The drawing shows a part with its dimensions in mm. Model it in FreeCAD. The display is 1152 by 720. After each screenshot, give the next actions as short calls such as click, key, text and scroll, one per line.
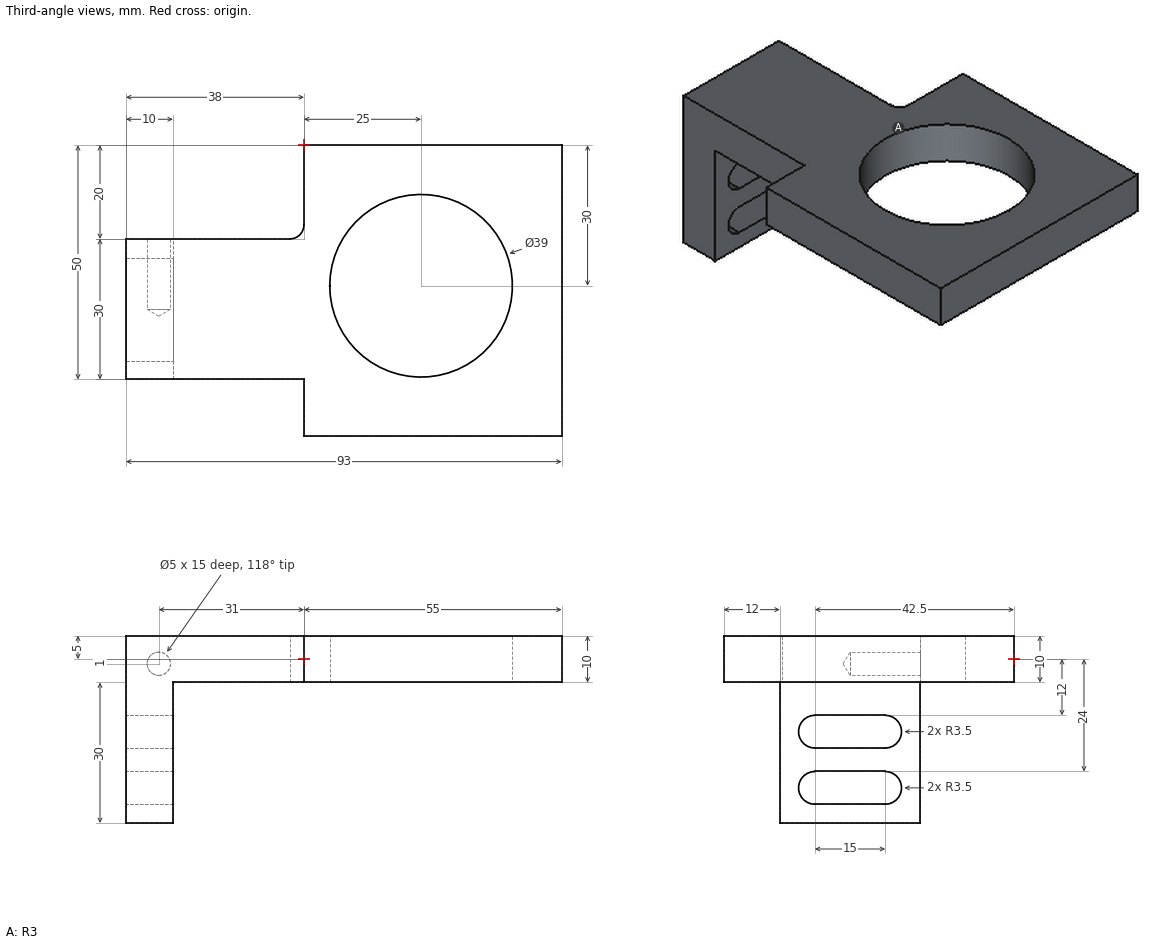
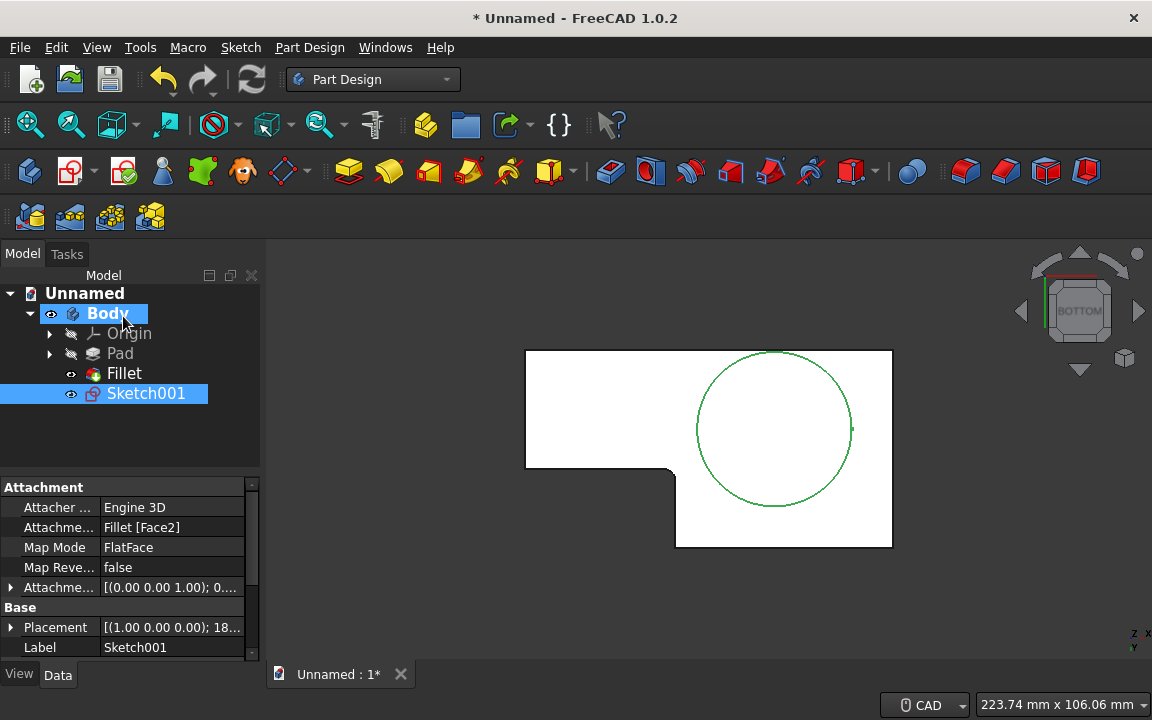
click(612, 172)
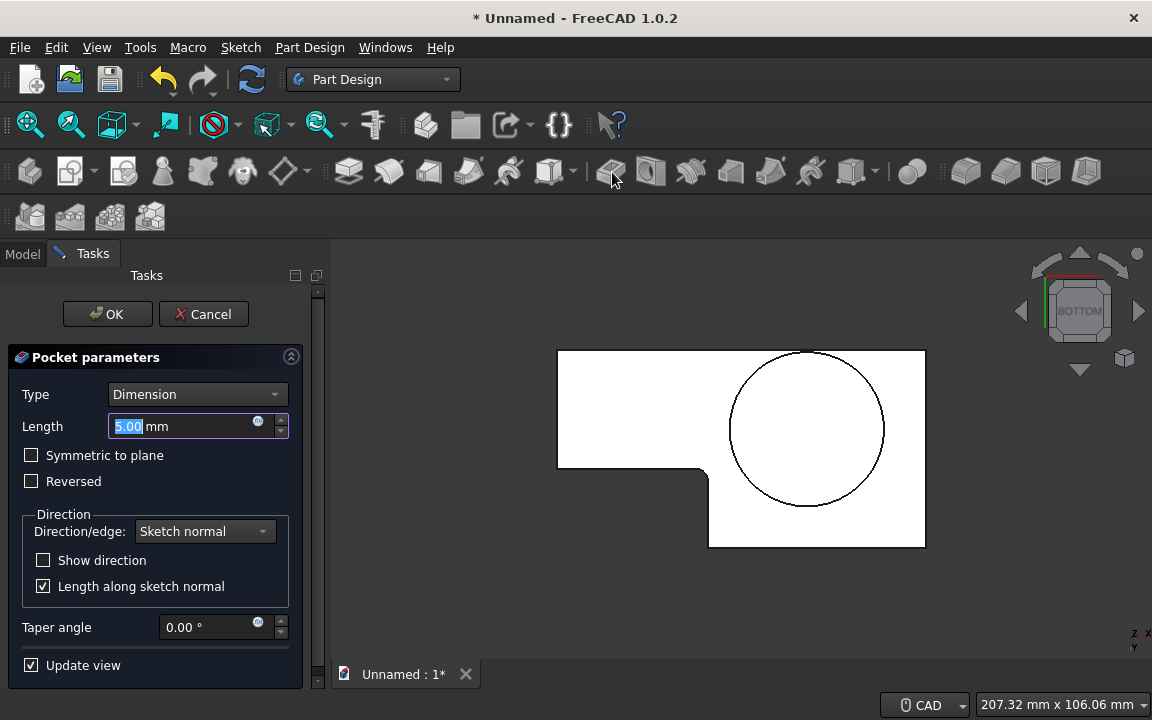
click(198, 394)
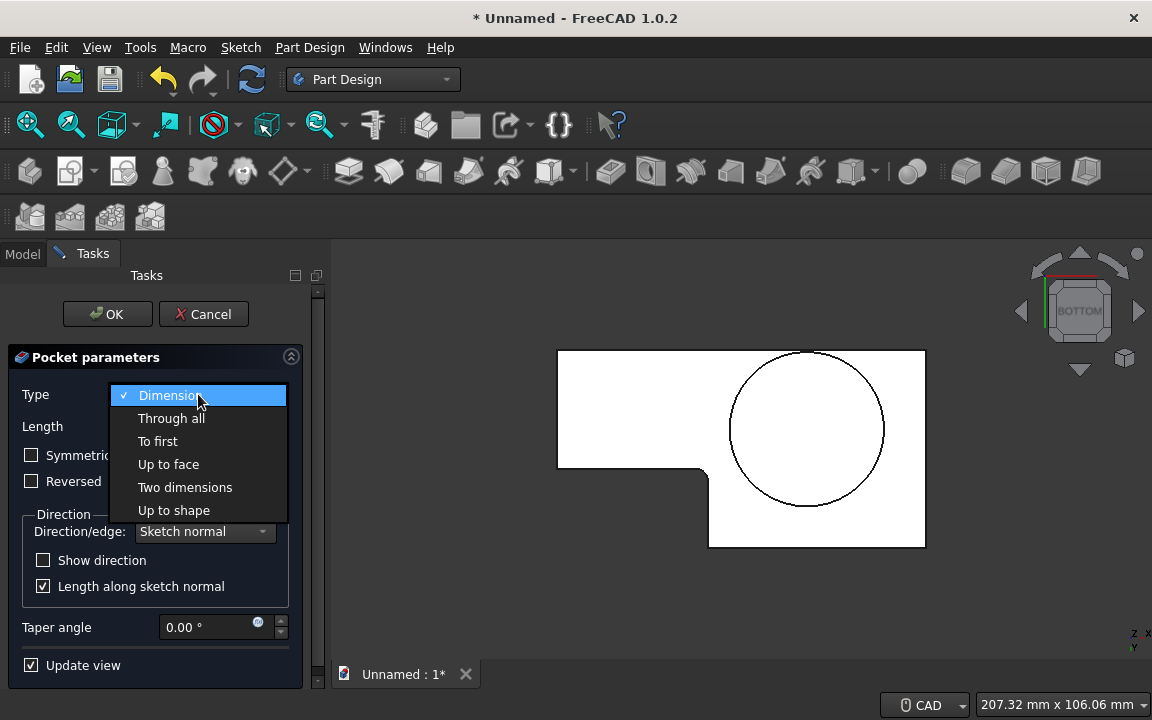
click(198, 442)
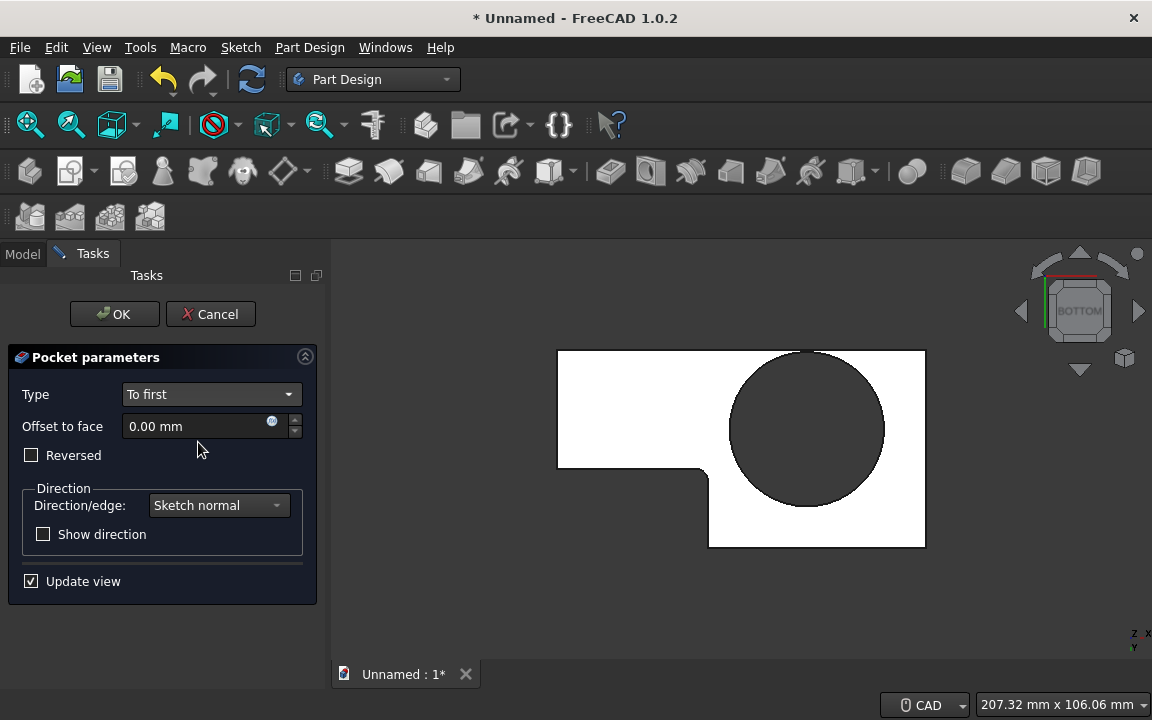
click(115, 314)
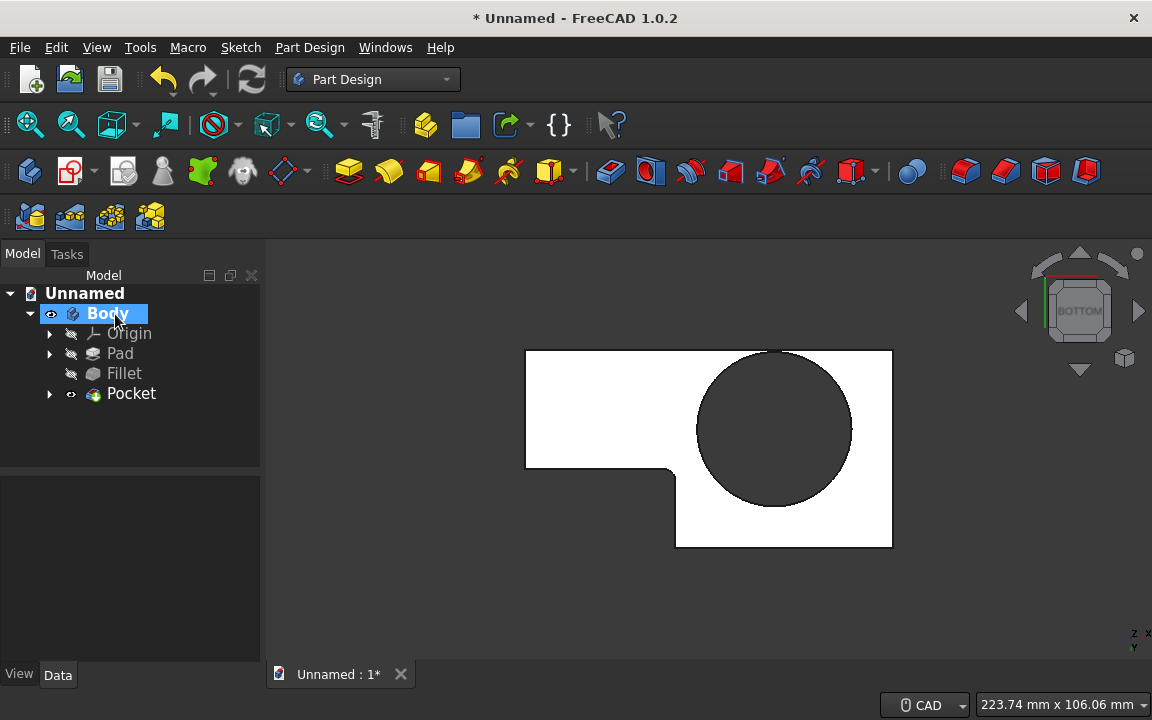
click(604, 420)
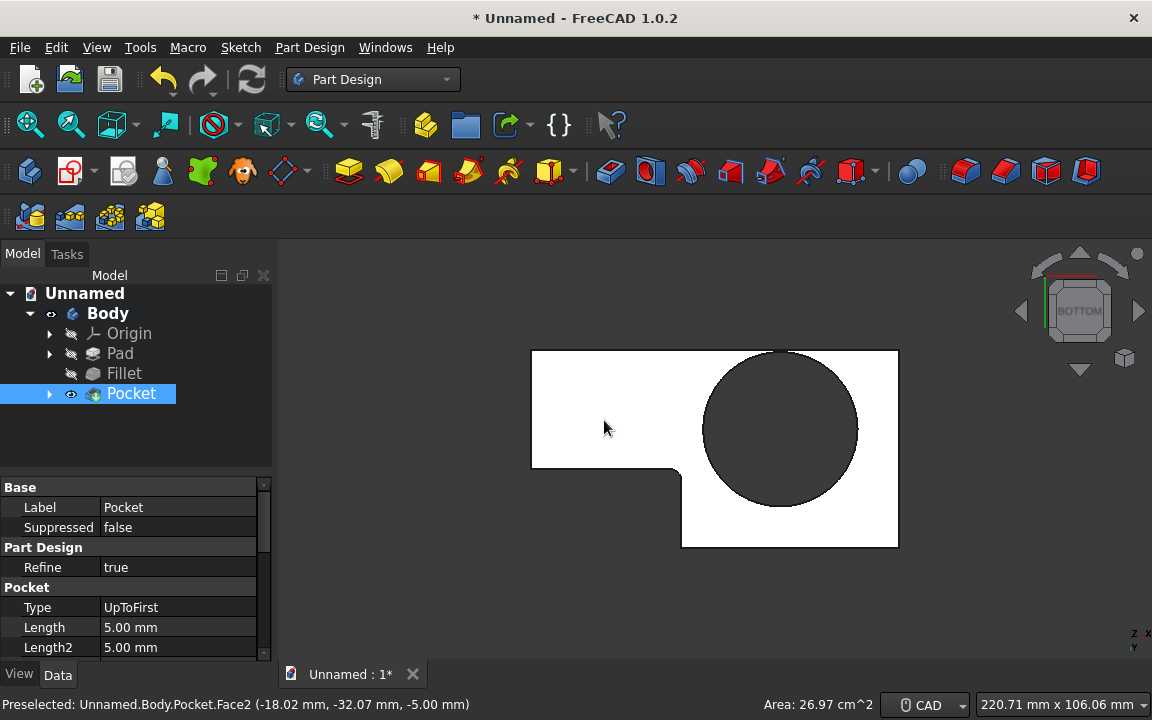
click(70, 172)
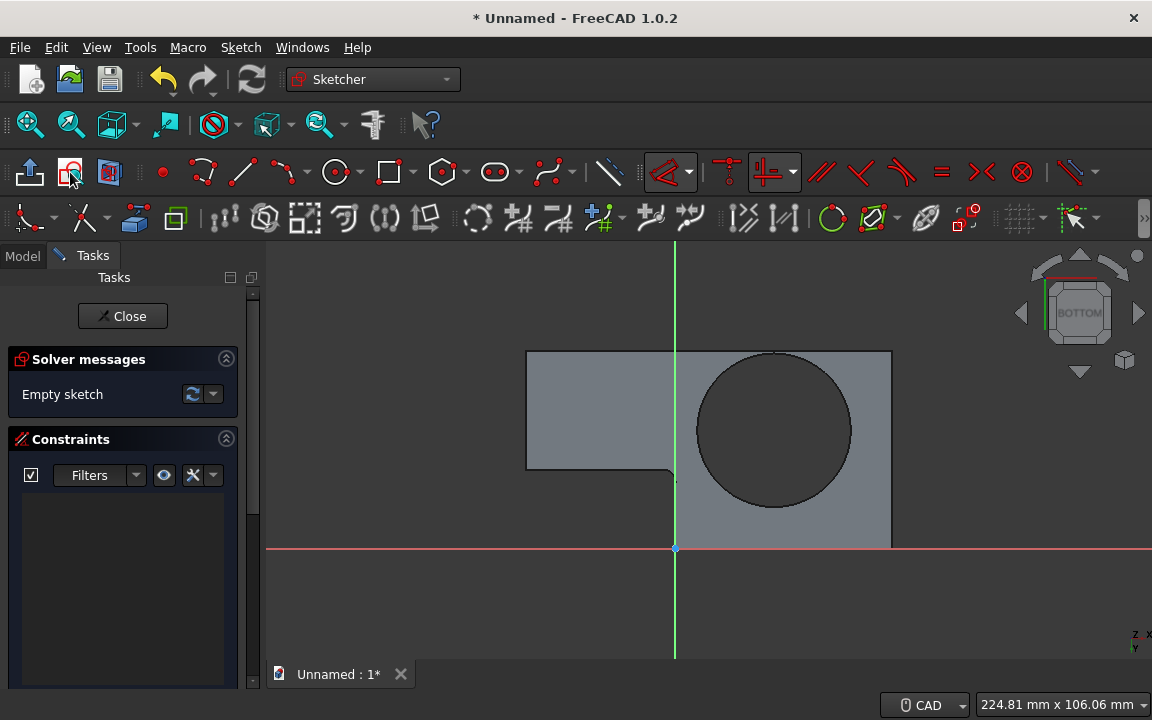
key(g)
key(r)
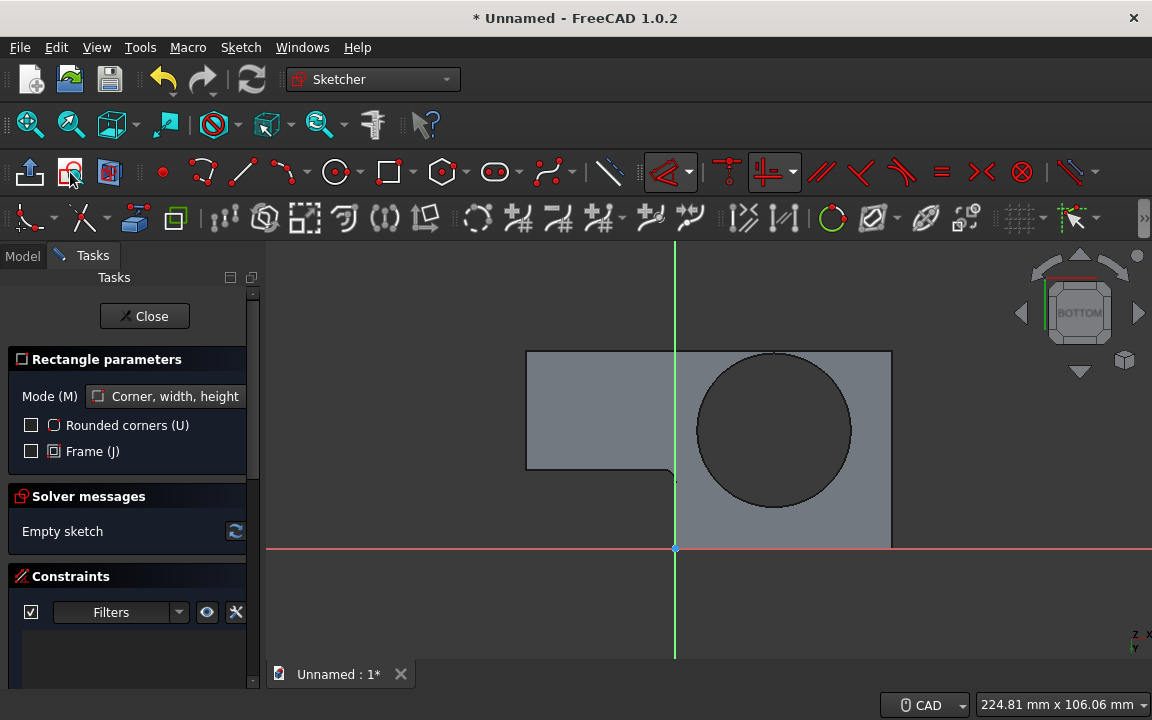
click(526, 351)
move(565, 470)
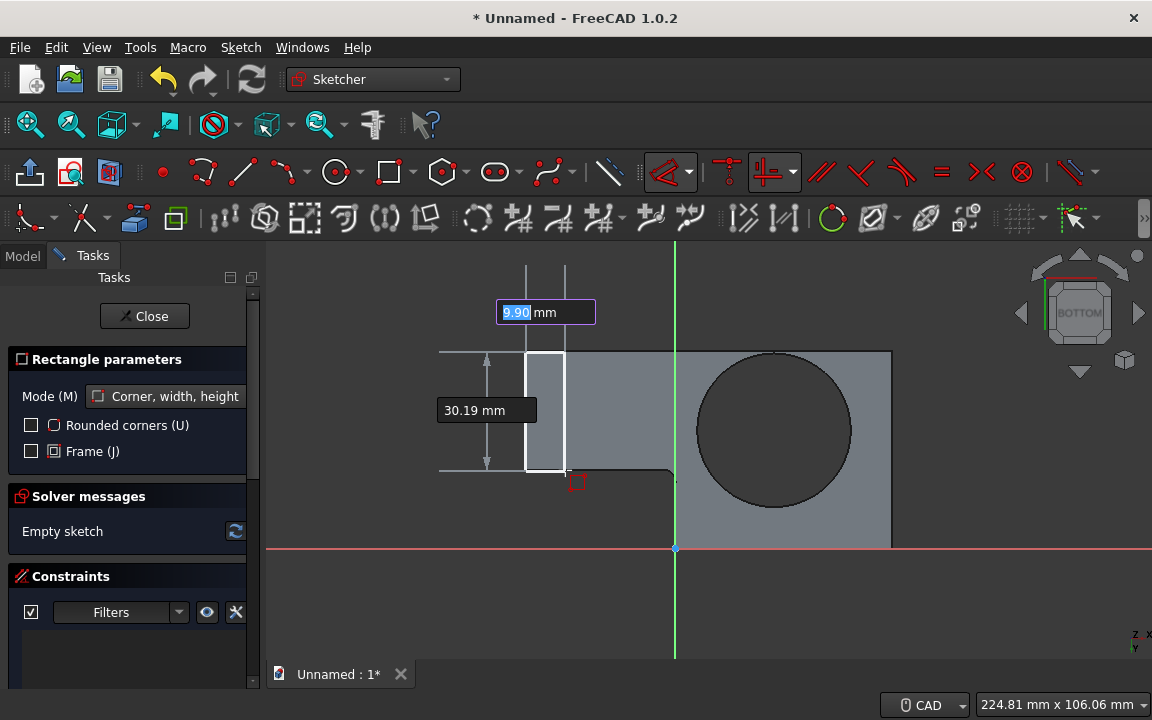
text(10)
key(Tab)
text(30)
key(Return)
key(Escape)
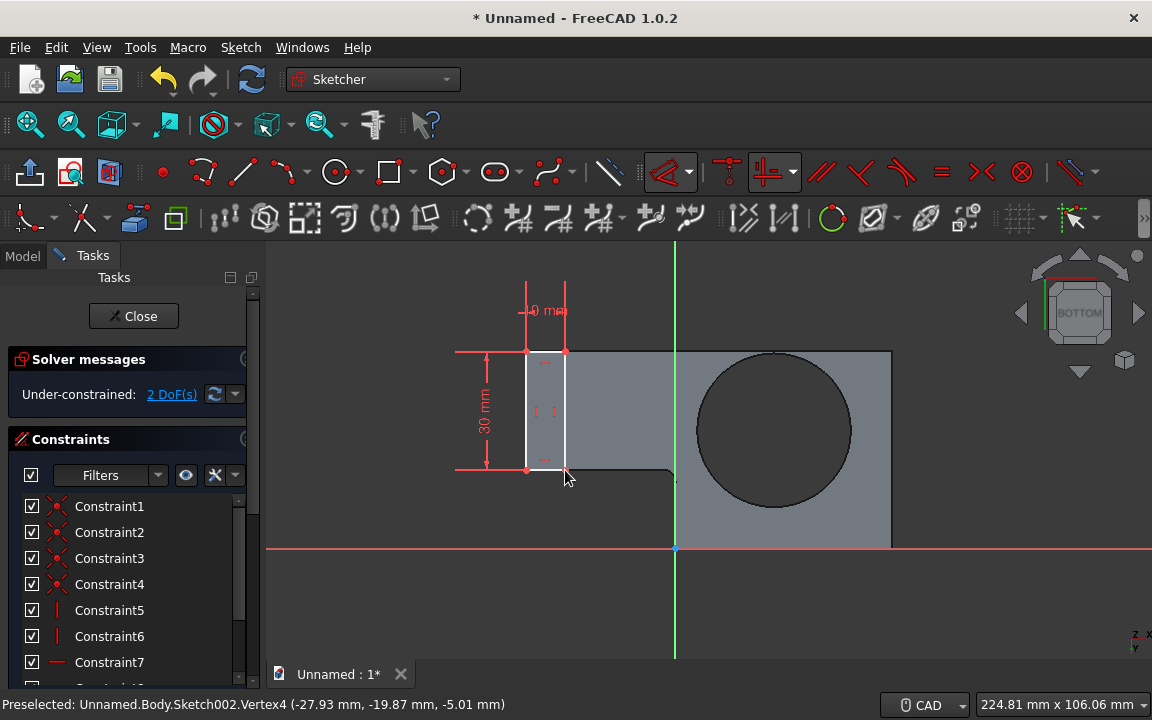
click(526, 352)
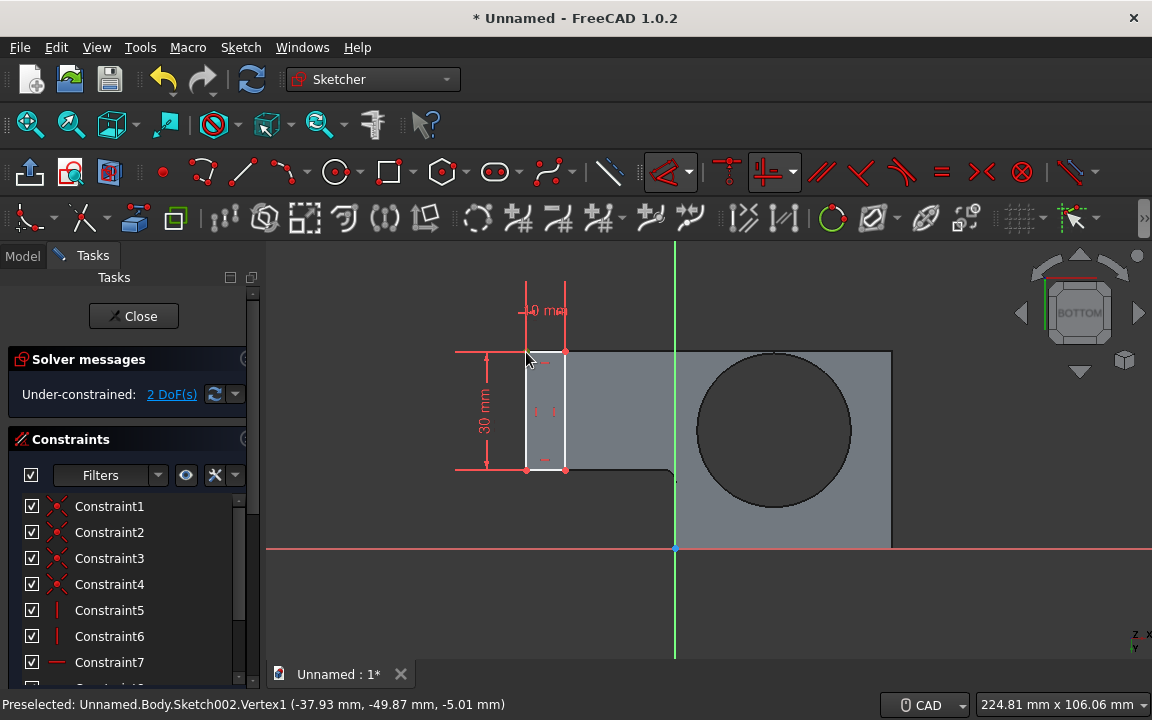
key(l)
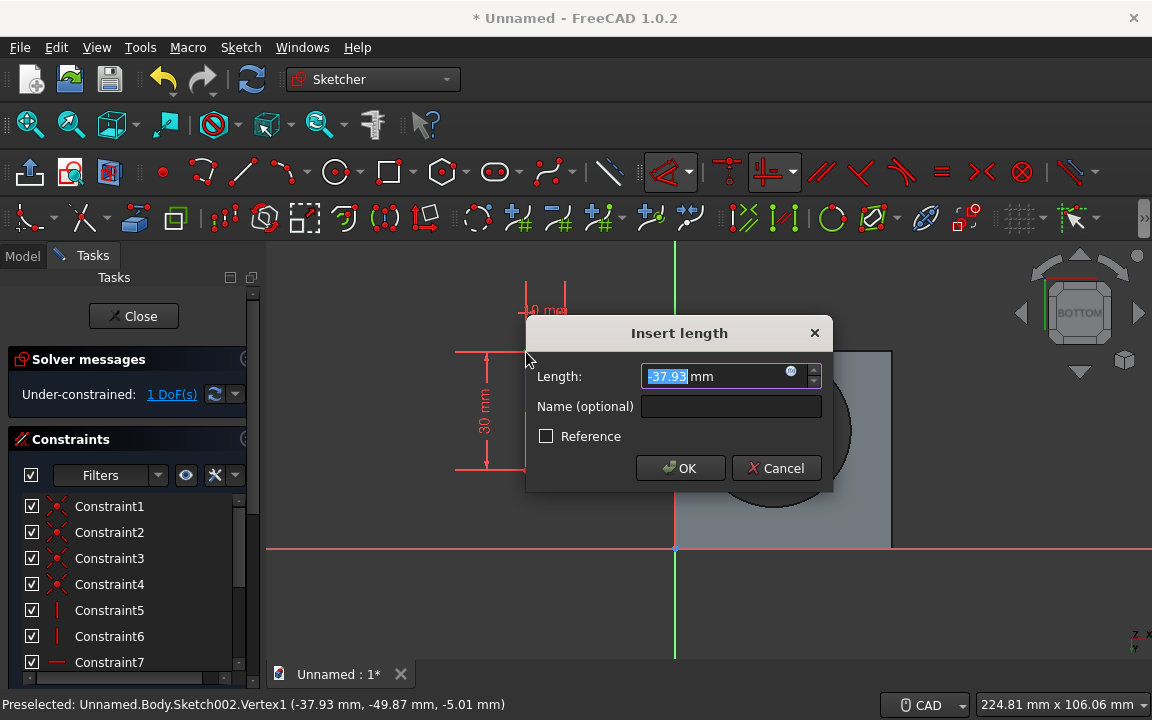
text(-38)
key(Return)